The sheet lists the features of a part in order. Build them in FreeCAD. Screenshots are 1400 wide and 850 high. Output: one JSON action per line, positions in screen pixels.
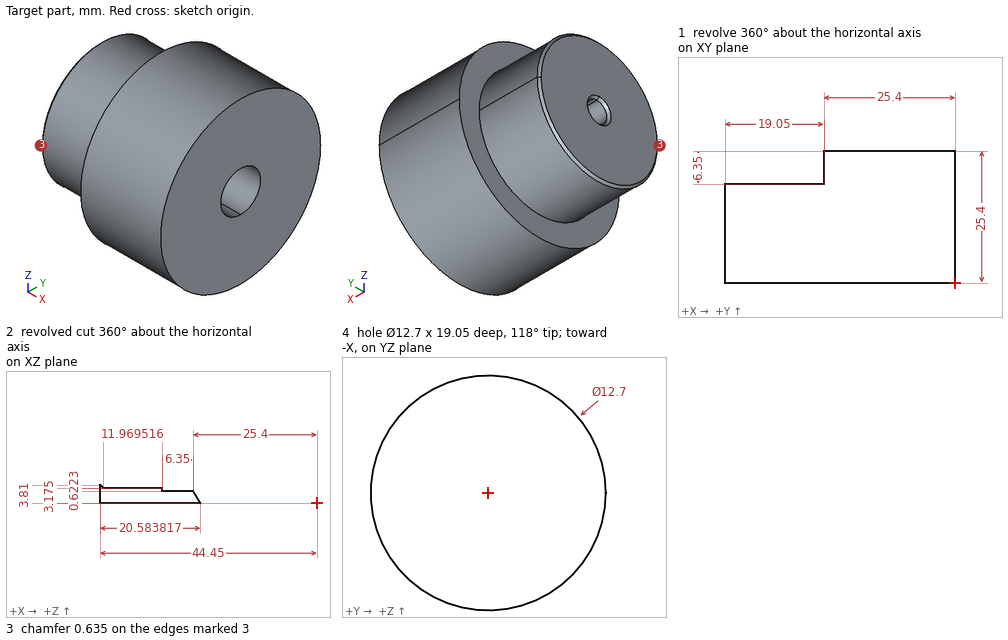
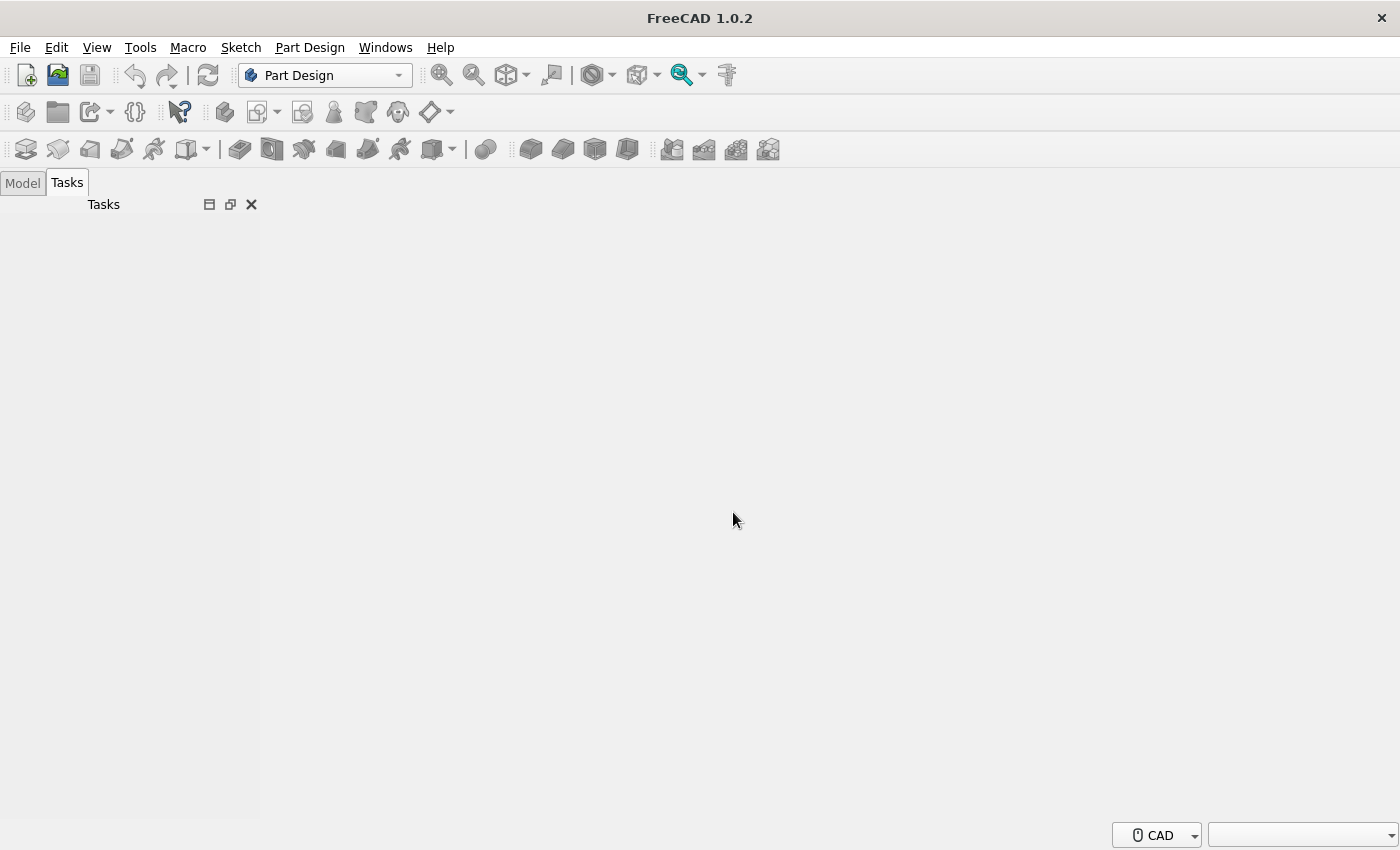
{"action": "left_click", "coordinate": [26, 76]}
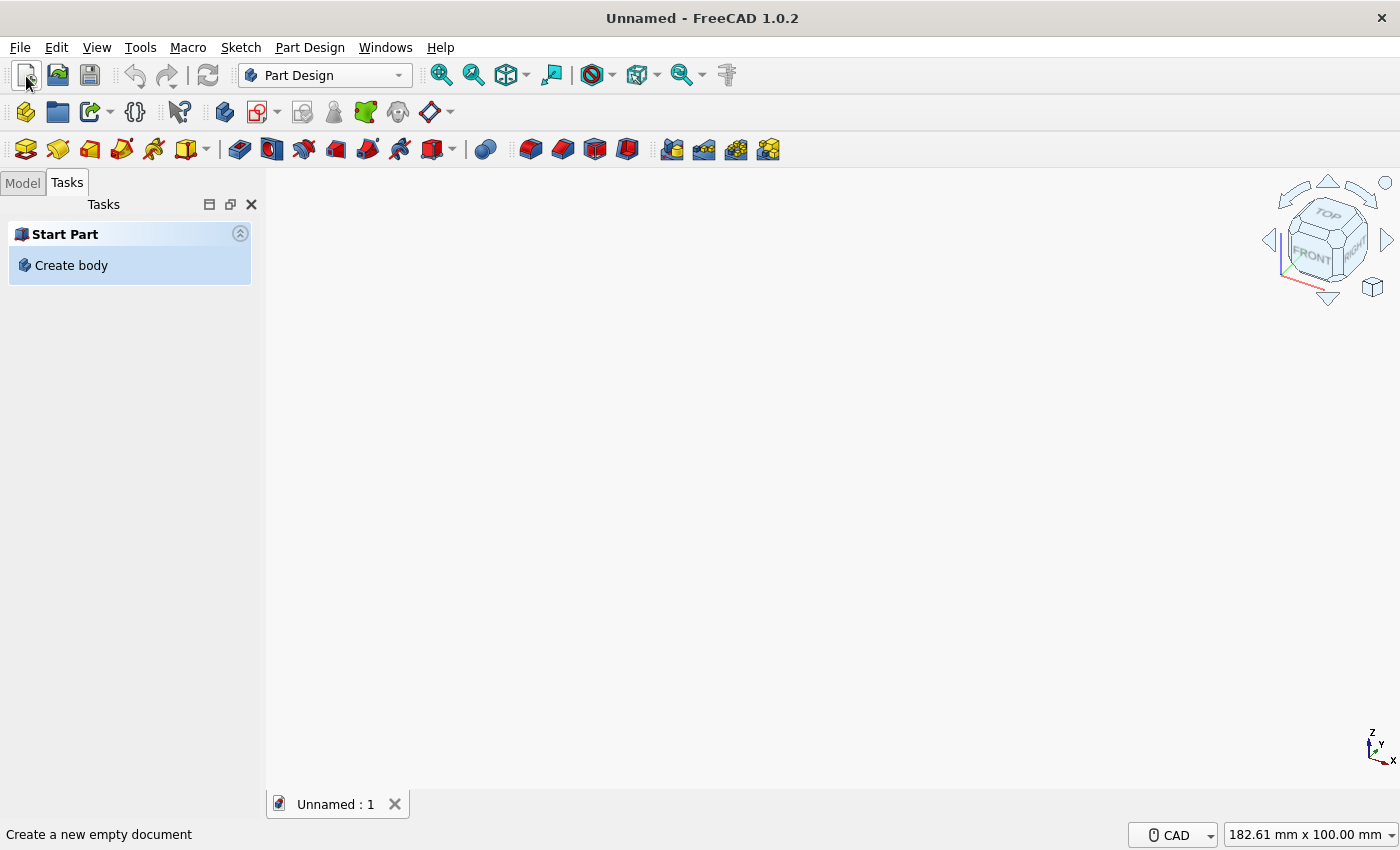
{"action": "left_click", "coordinate": [258, 112]}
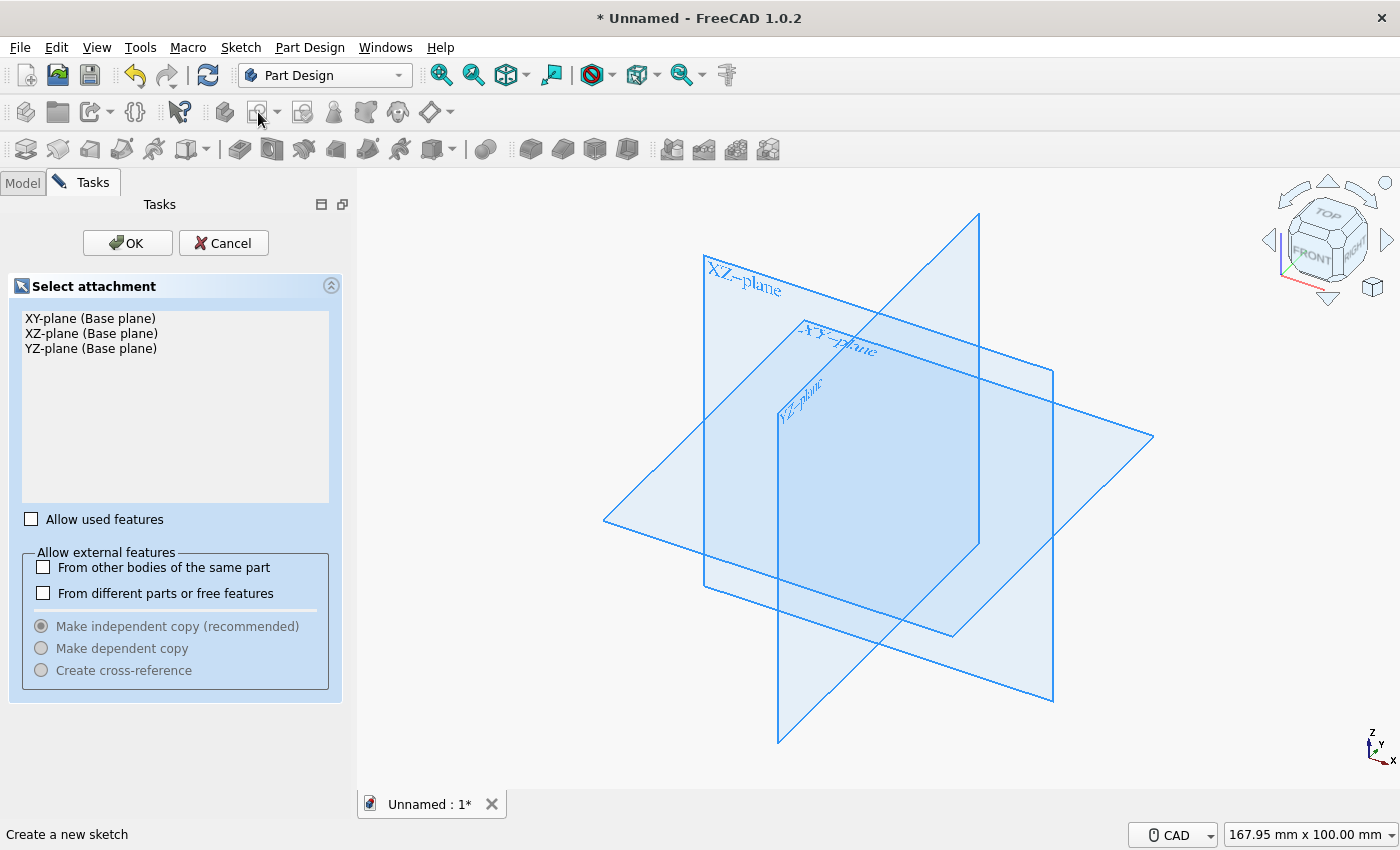
{"action": "left_click", "coordinate": [82, 318]}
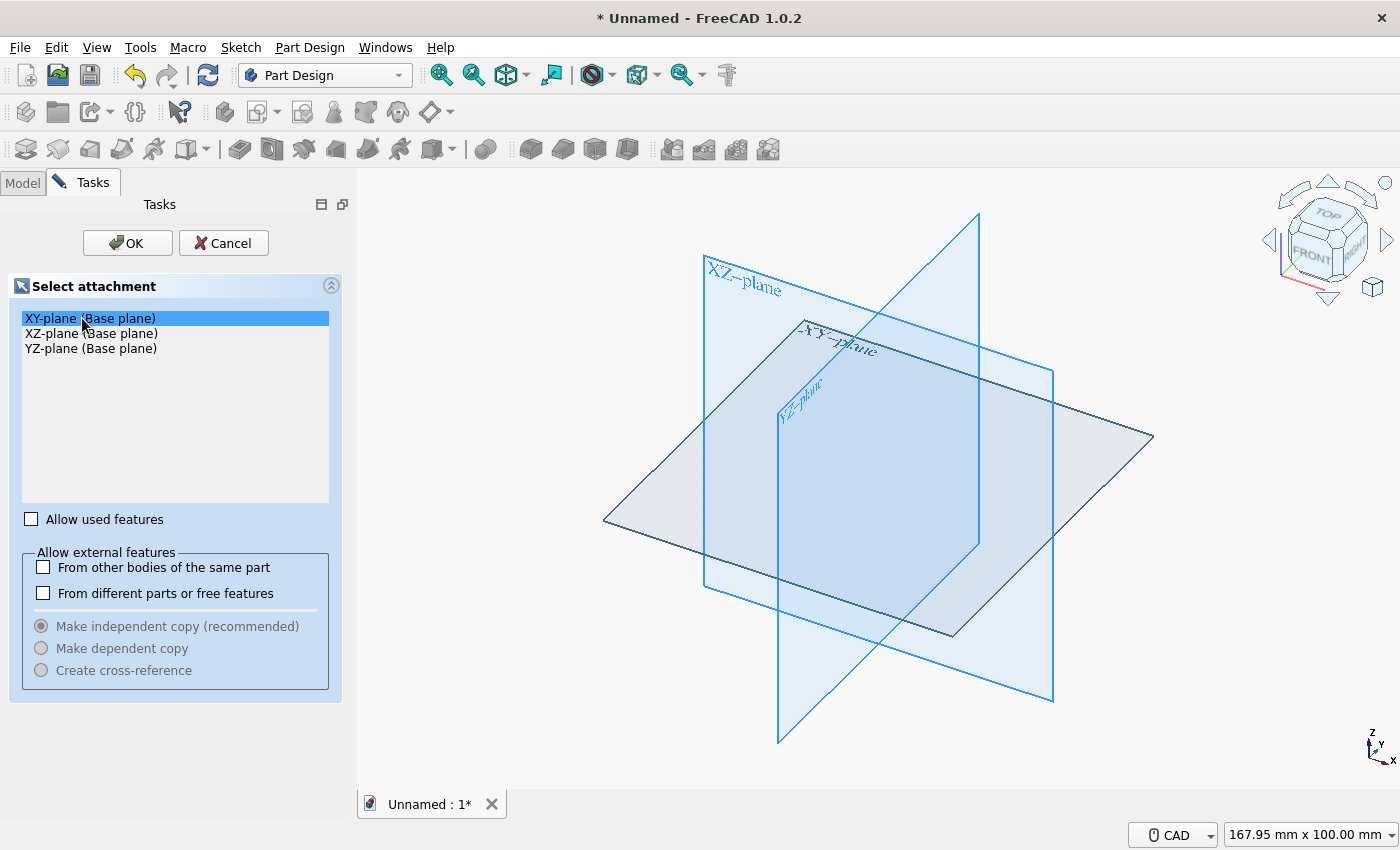
{"action": "left_click", "coordinate": [128, 243]}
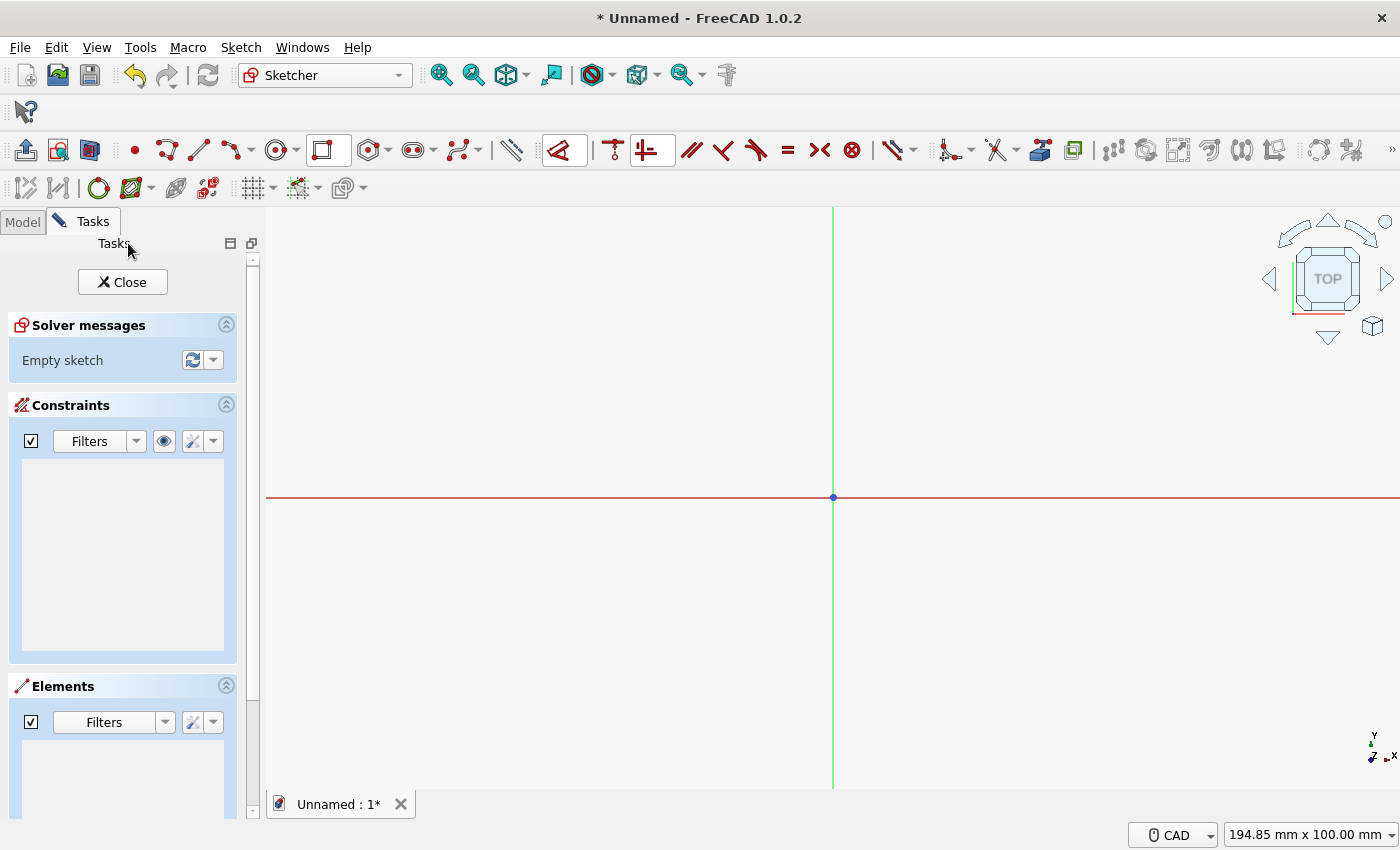
{"action": "scroll", "coordinate": [668, 381], "scroll_direction": "up", "scroll_amount": 5}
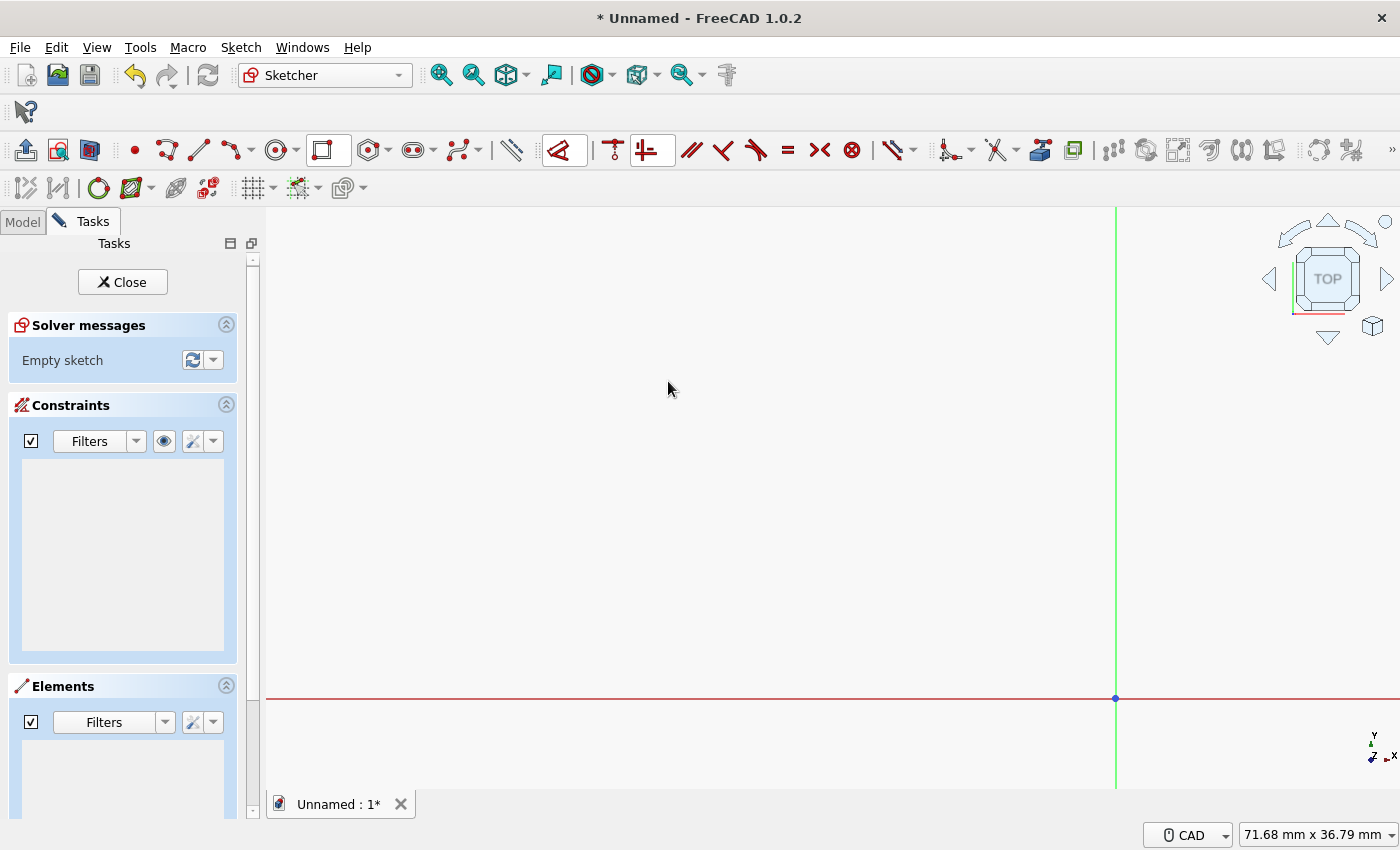
{"action": "left_click", "coordinate": [168, 150]}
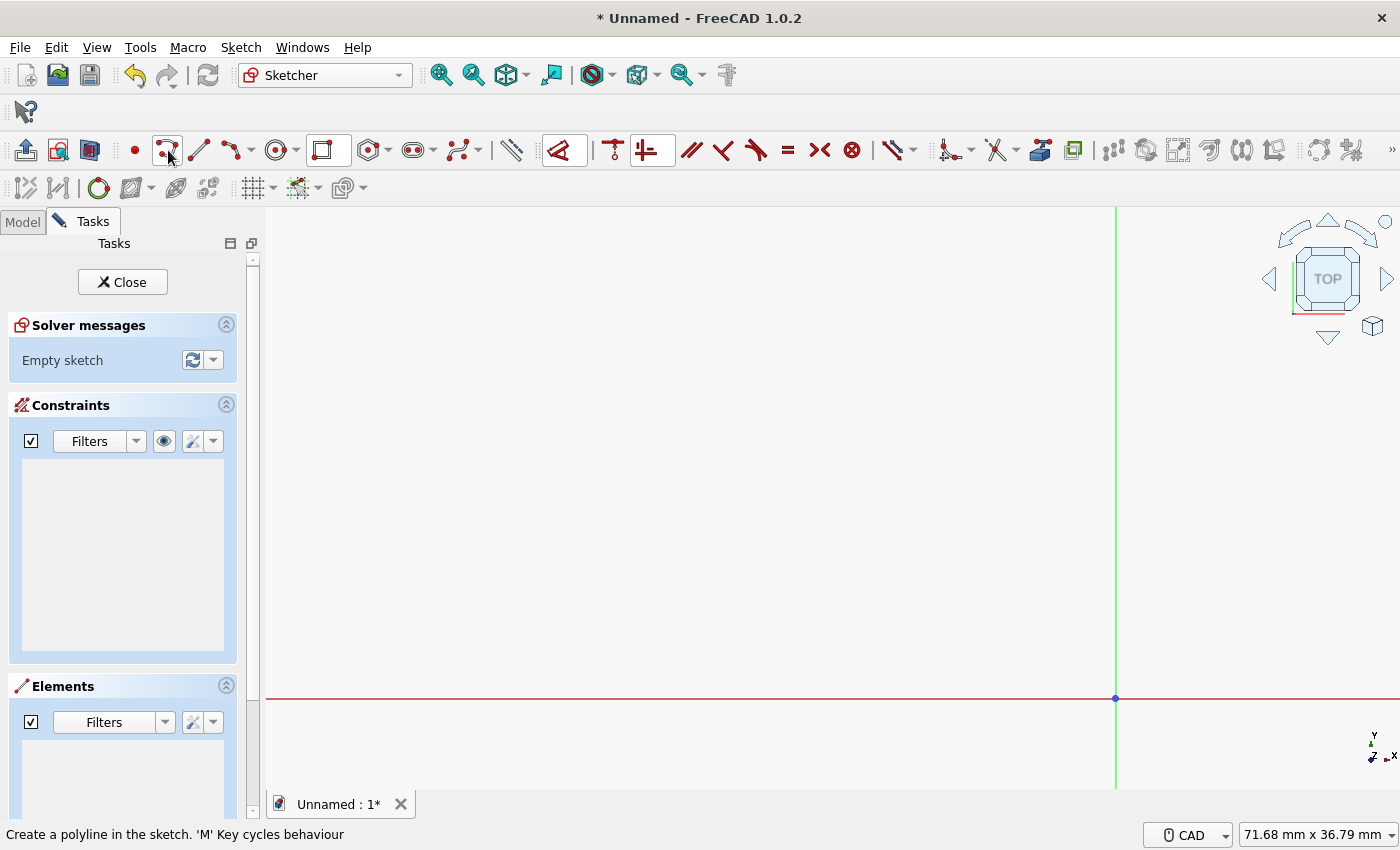
{"action": "left_click", "coordinate": [1116, 699]}
{"action": "left_click", "coordinate": [1107, 297]}
{"action": "left_click", "coordinate": [714, 297]}
{"action": "left_click", "coordinate": [714, 397]}
{"action": "left_click", "coordinate": [413, 397]}
{"action": "left_click", "coordinate": [413, 690]}
{"action": "left_click", "coordinate": [1116, 699]}
{"action": "key", "text": "Escape"}
{"action": "key", "text": "Escape"}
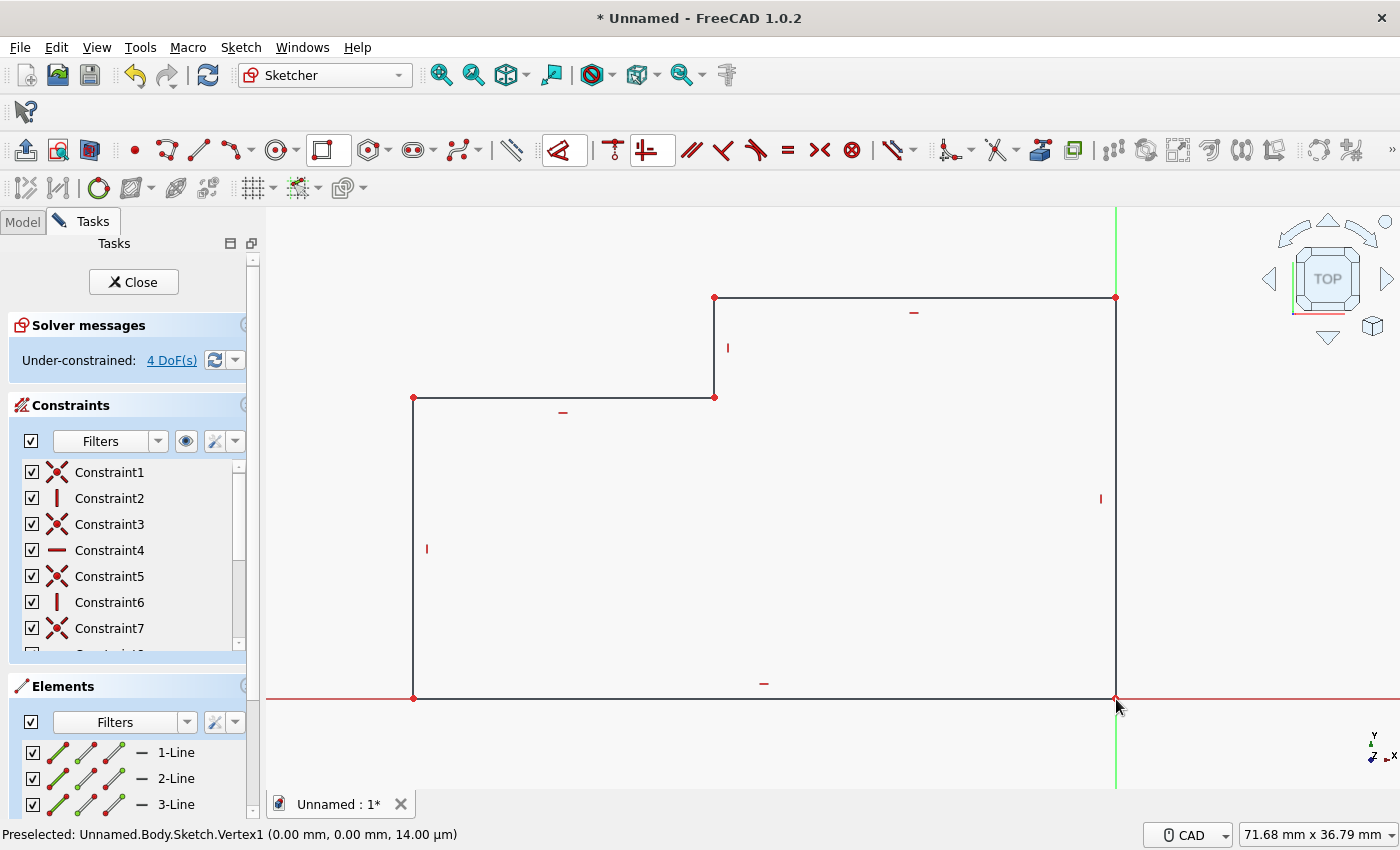
{"action": "left_click", "coordinate": [558, 150]}